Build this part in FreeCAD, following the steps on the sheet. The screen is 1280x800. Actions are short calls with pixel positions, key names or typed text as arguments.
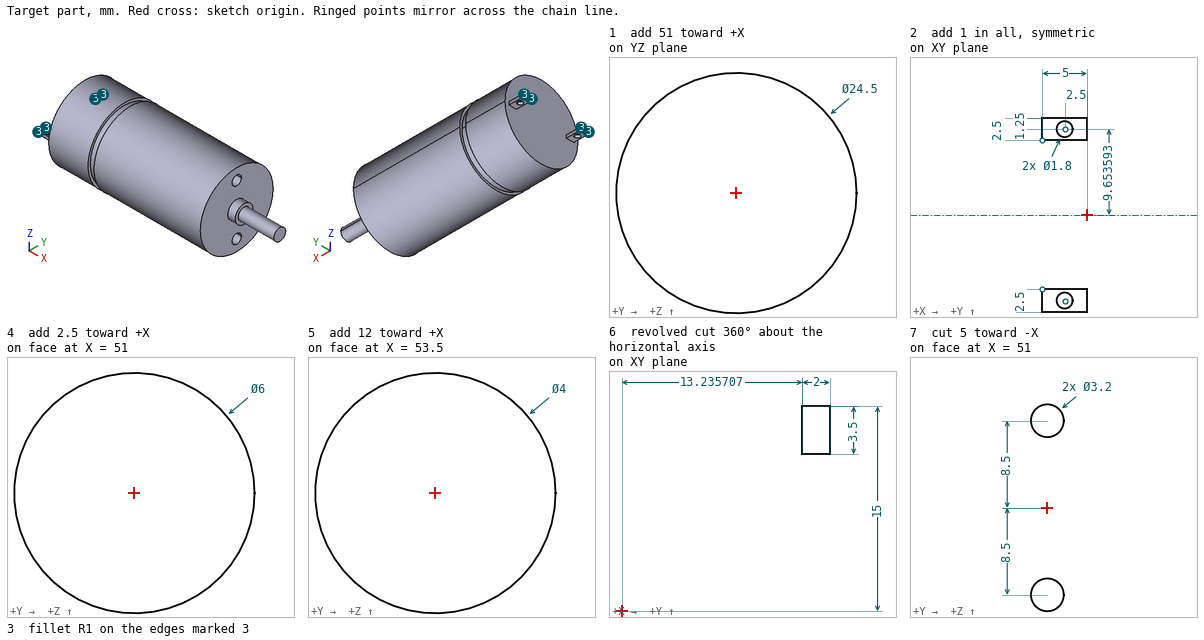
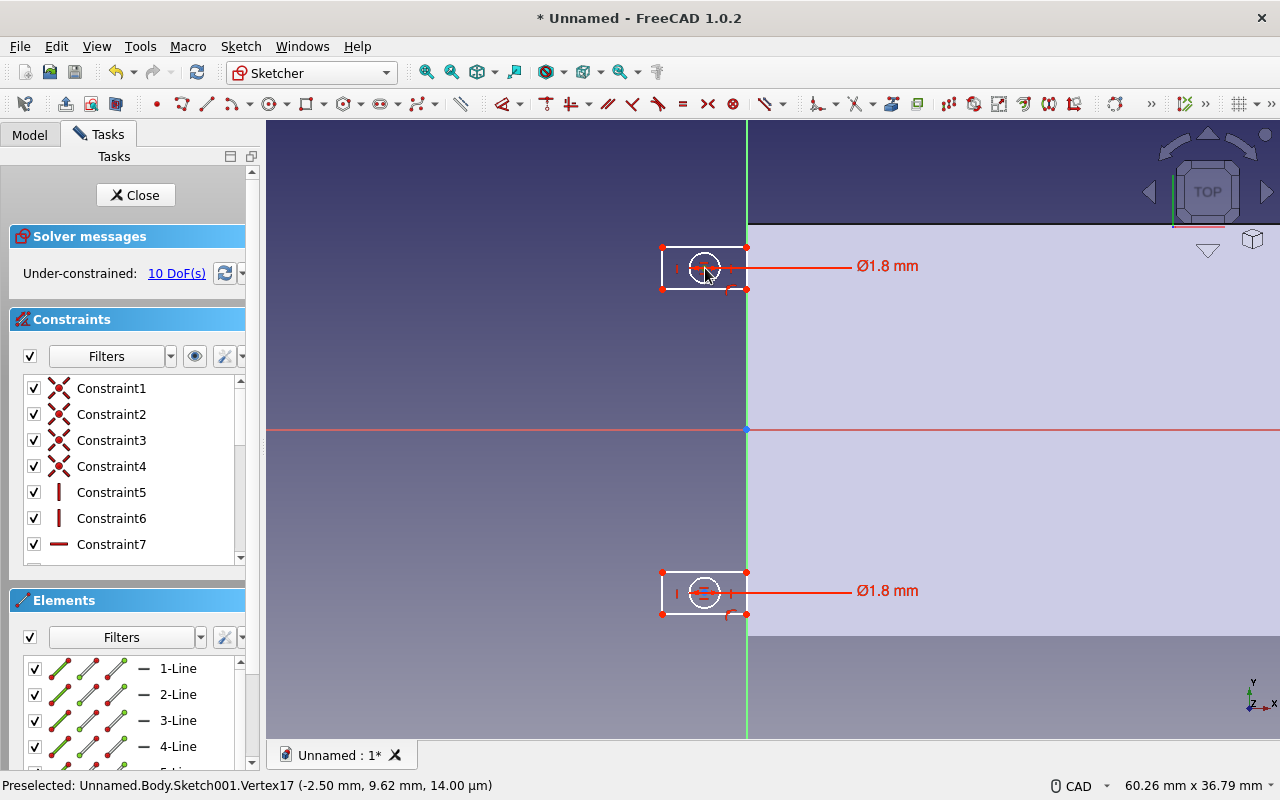
click(705, 593)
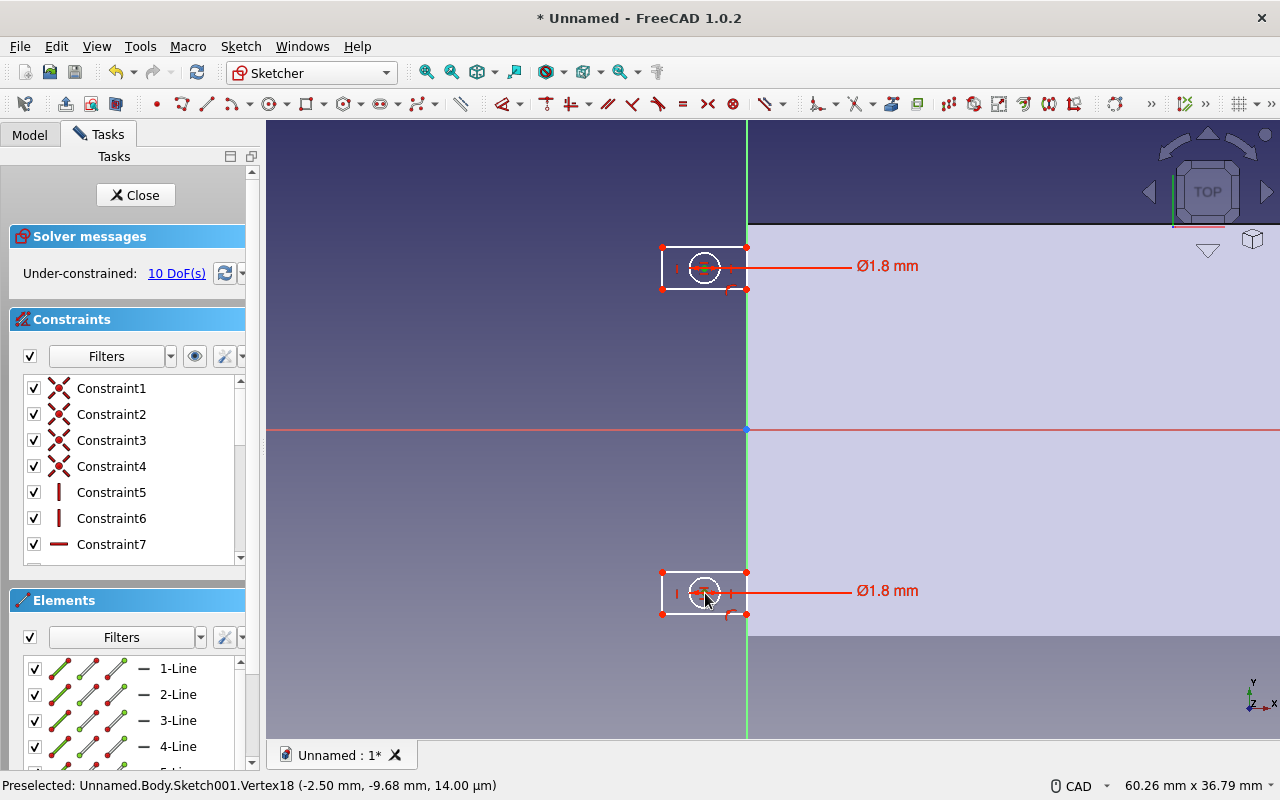
click(353, 430)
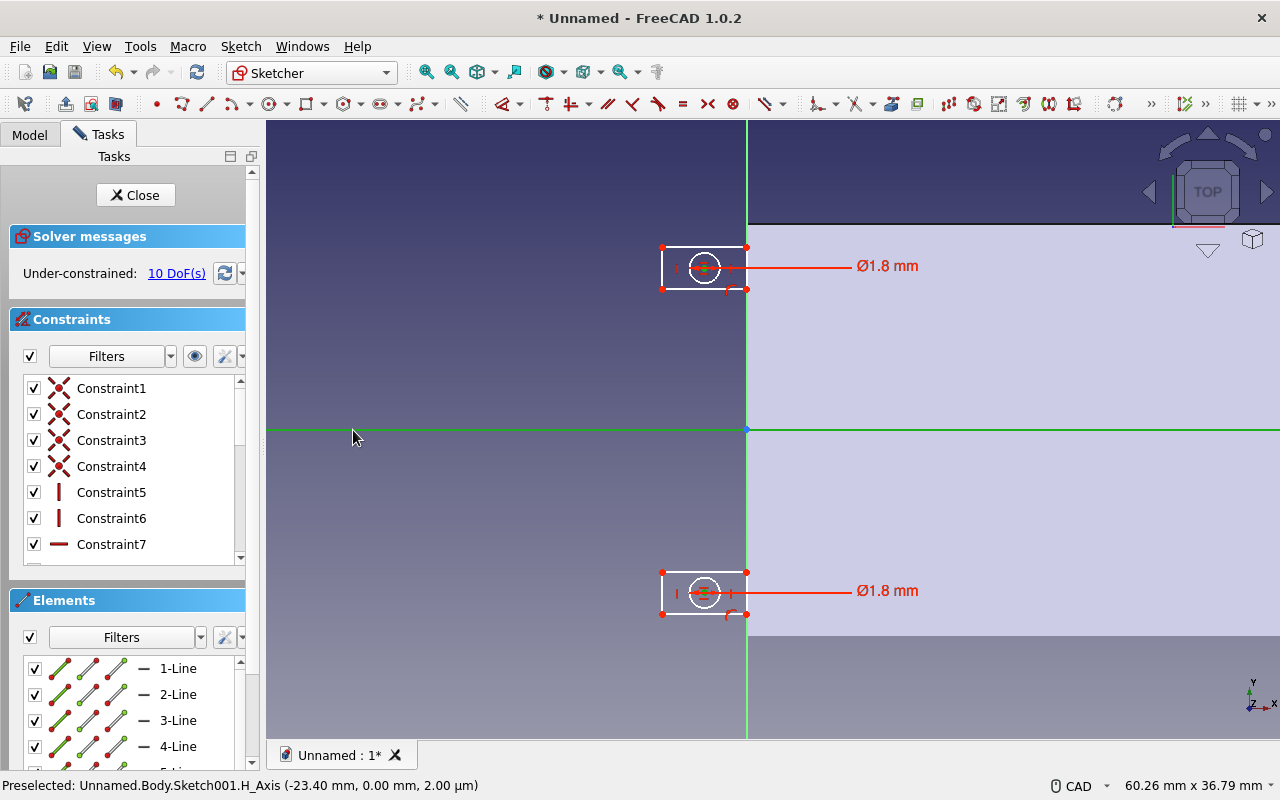
click(708, 104)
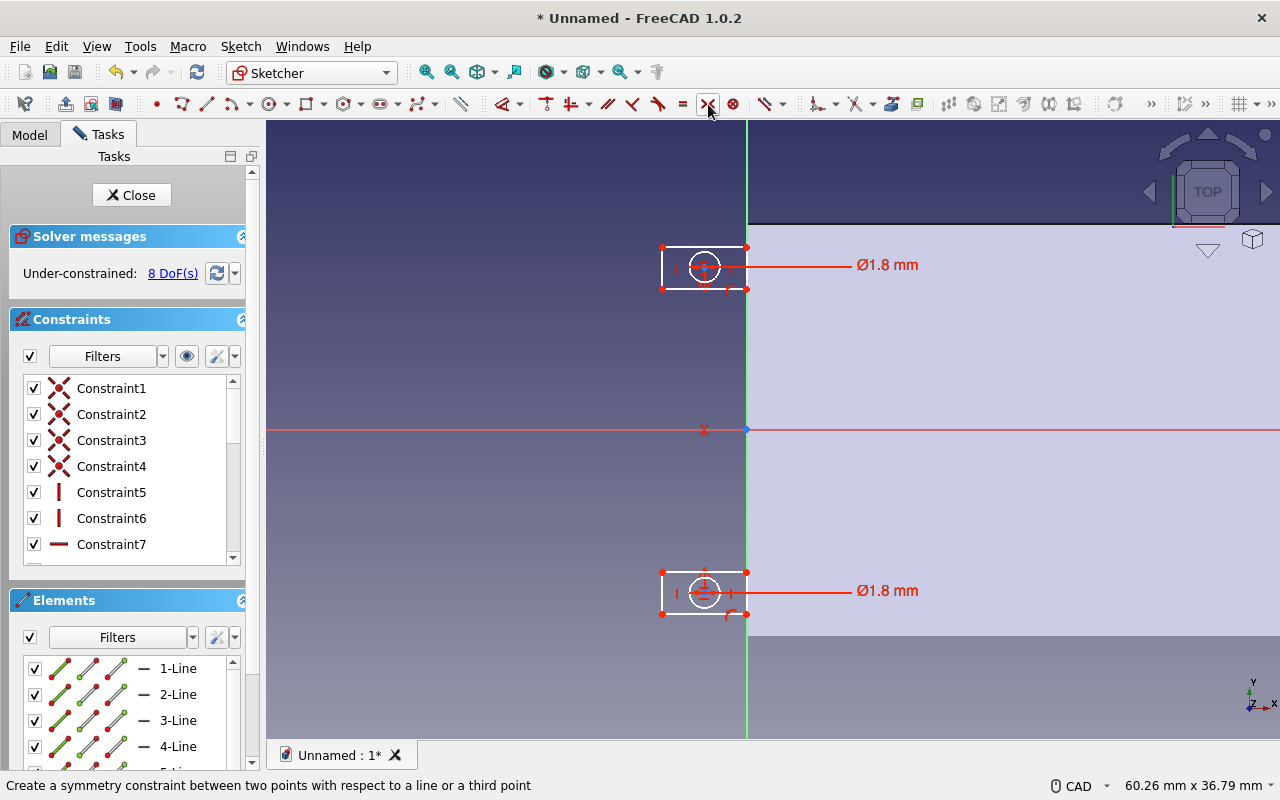
click(662, 289)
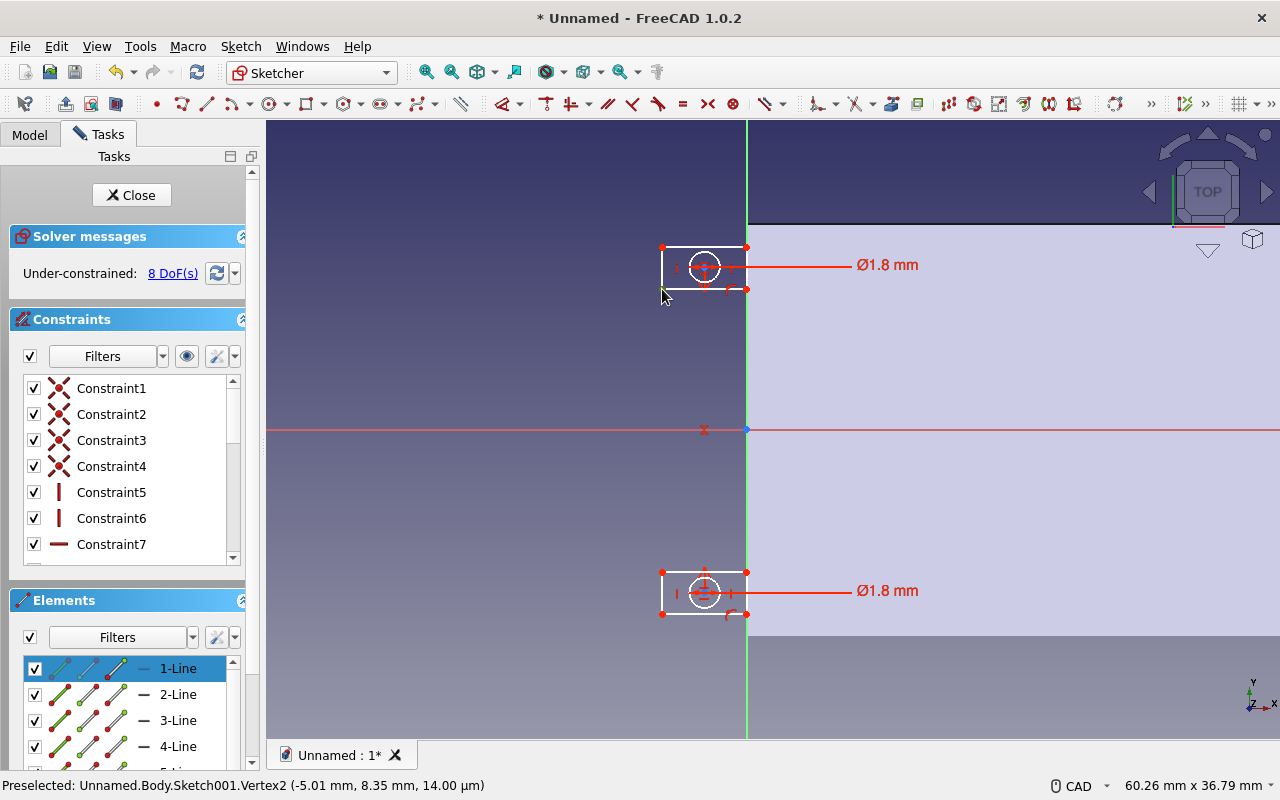
click(662, 572)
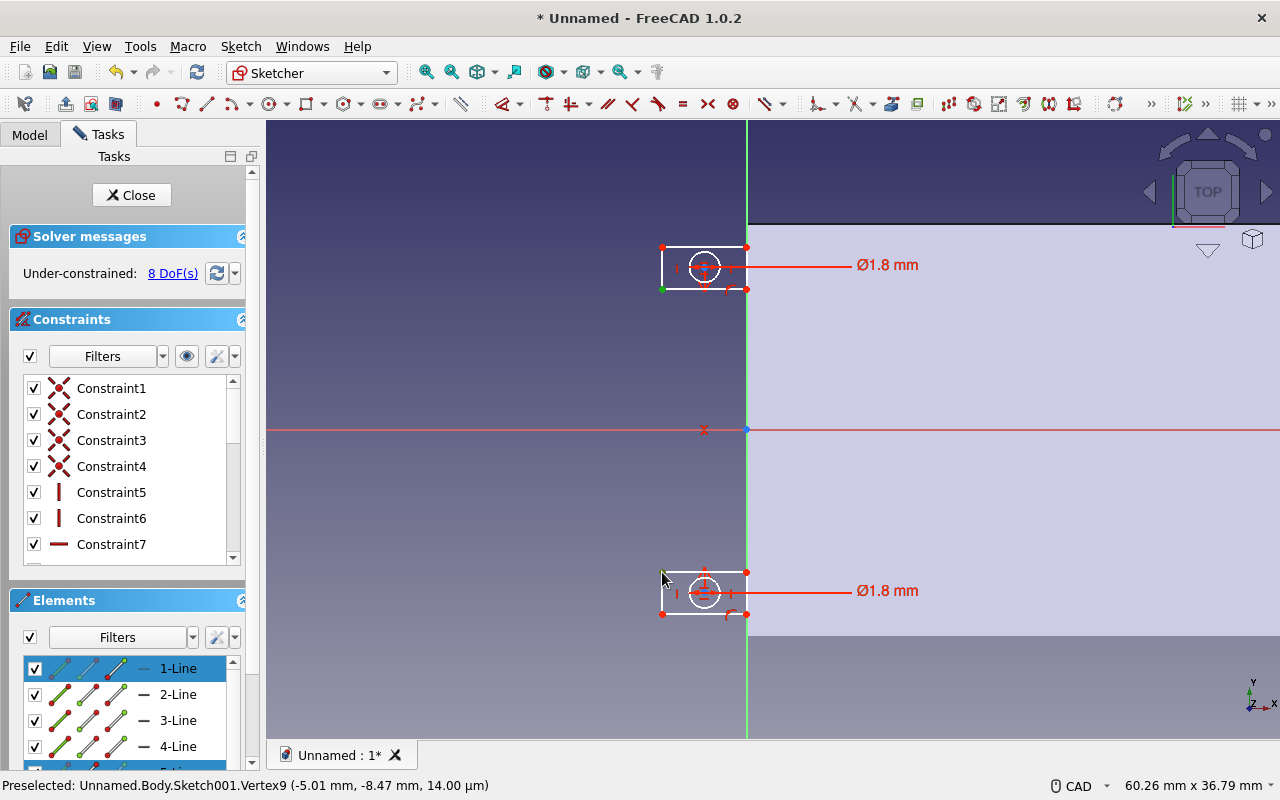
click(353, 430)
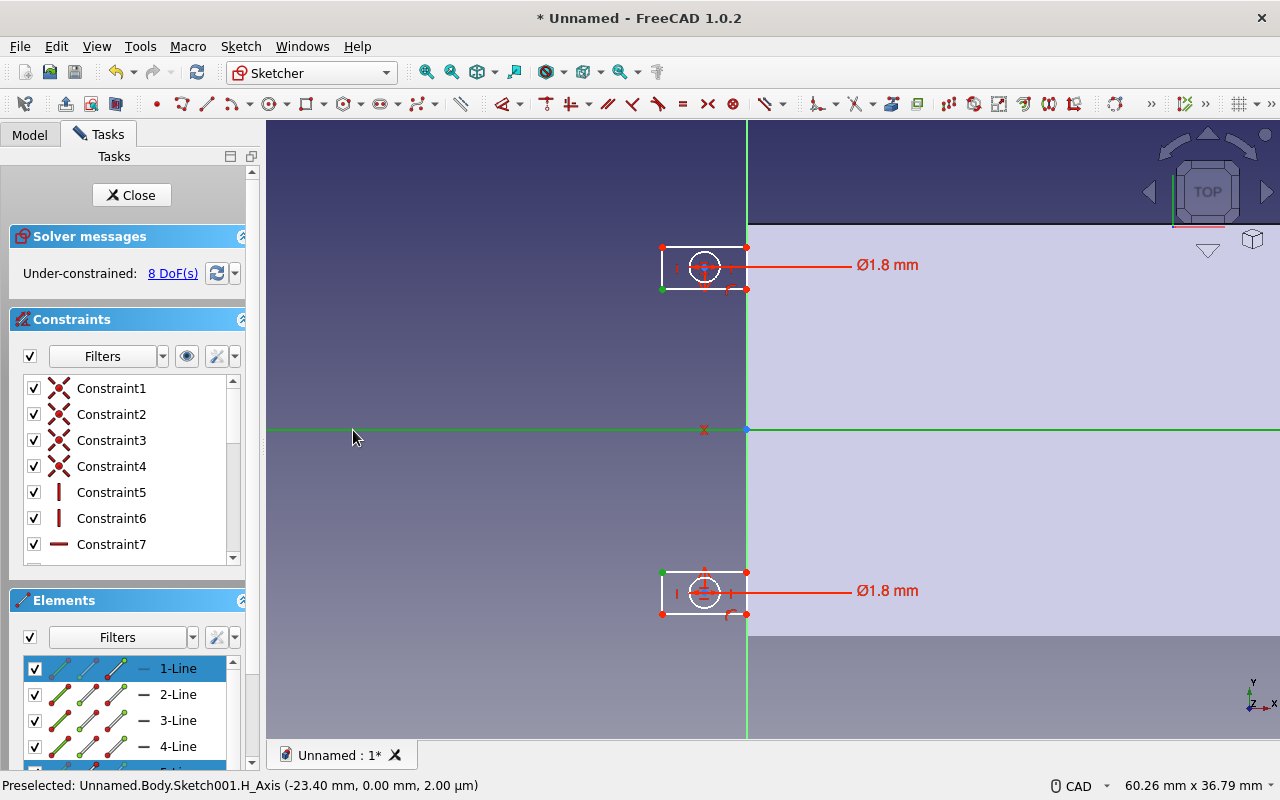
click(708, 104)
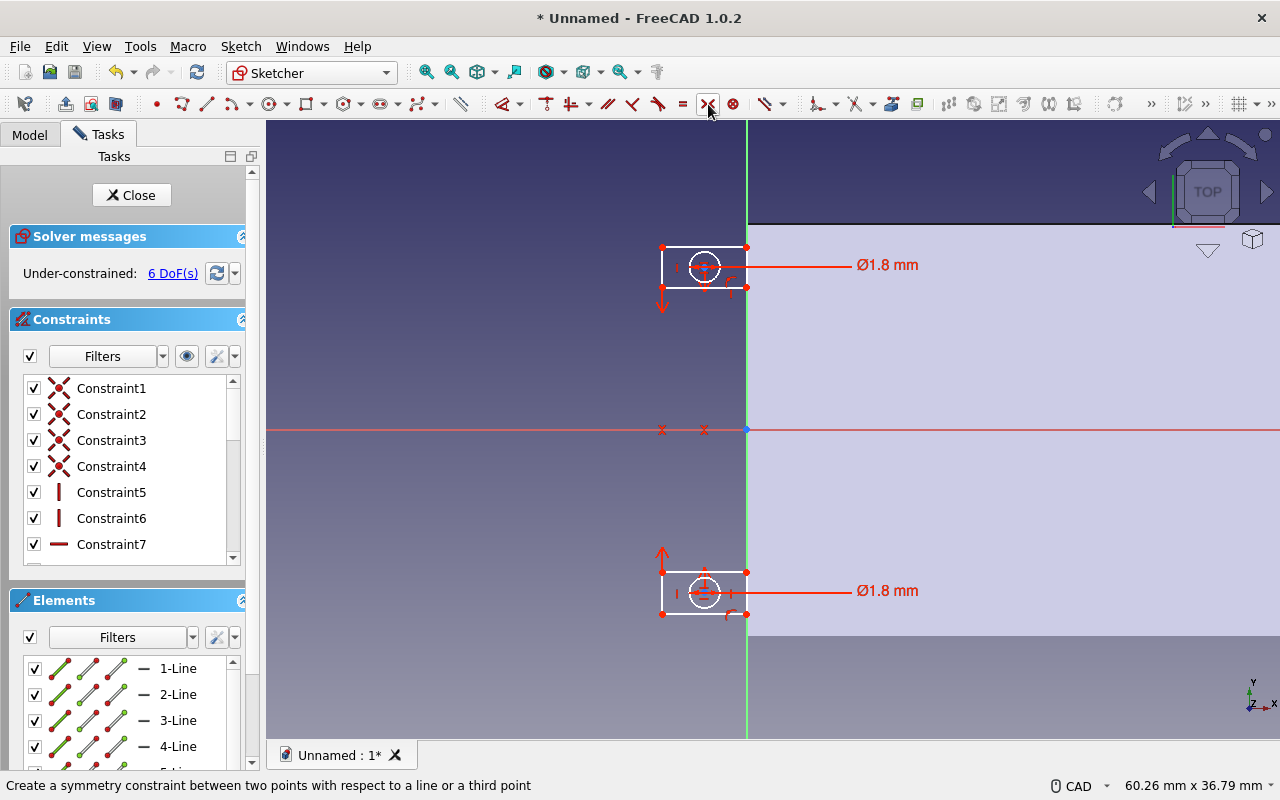
click(688, 288)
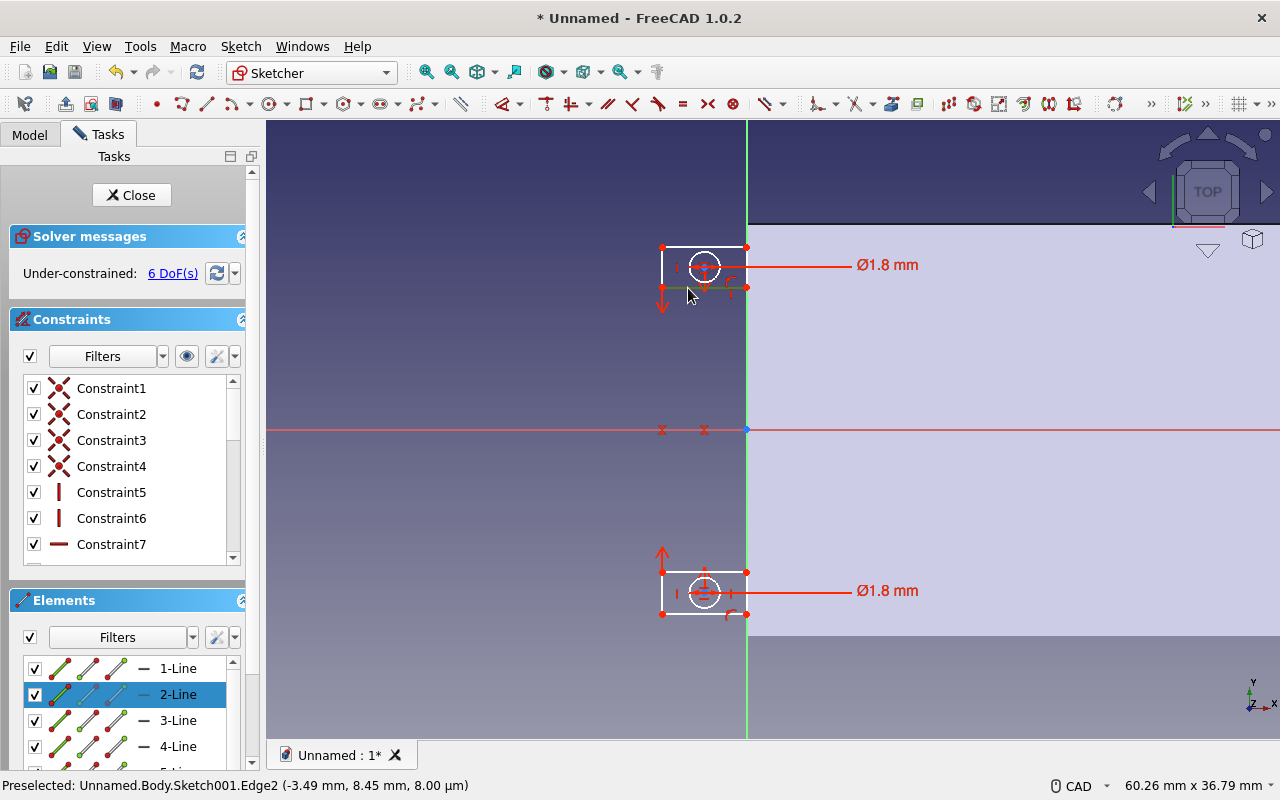
click(520, 104)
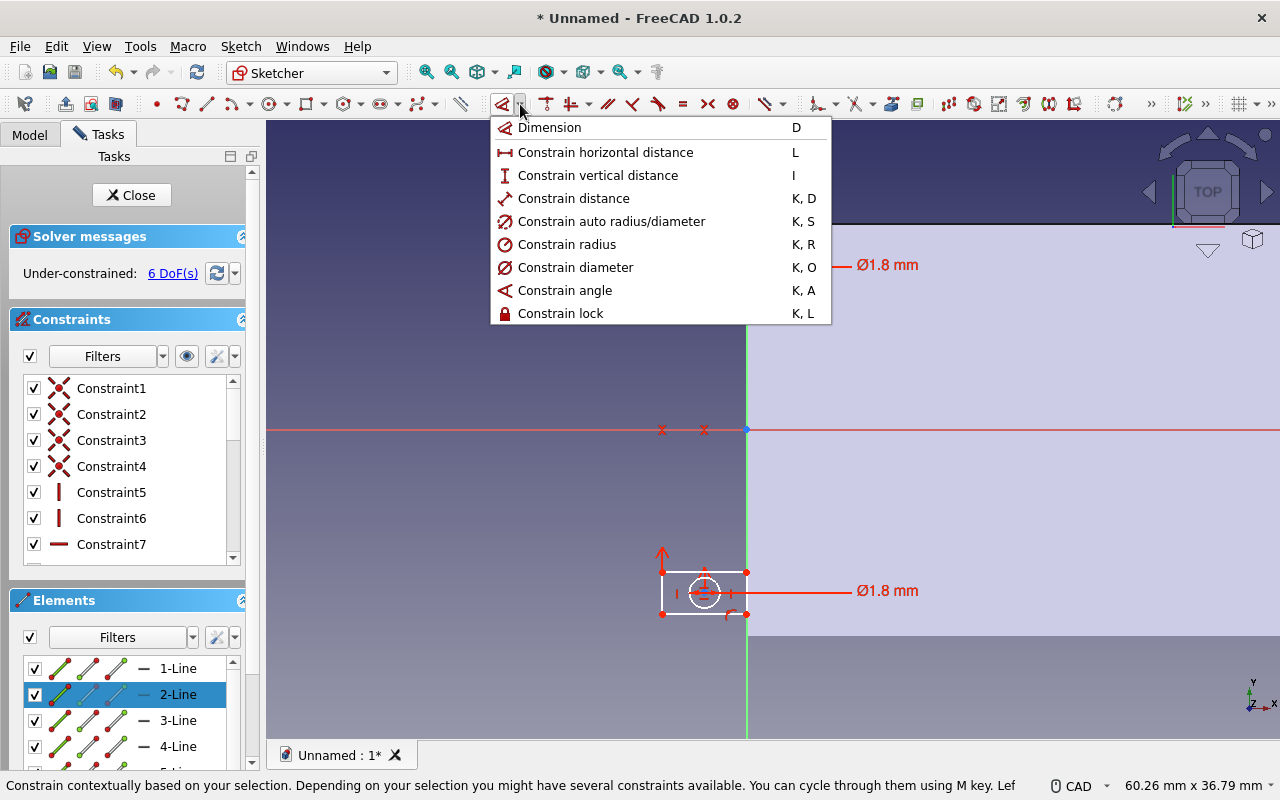
click(661, 152)